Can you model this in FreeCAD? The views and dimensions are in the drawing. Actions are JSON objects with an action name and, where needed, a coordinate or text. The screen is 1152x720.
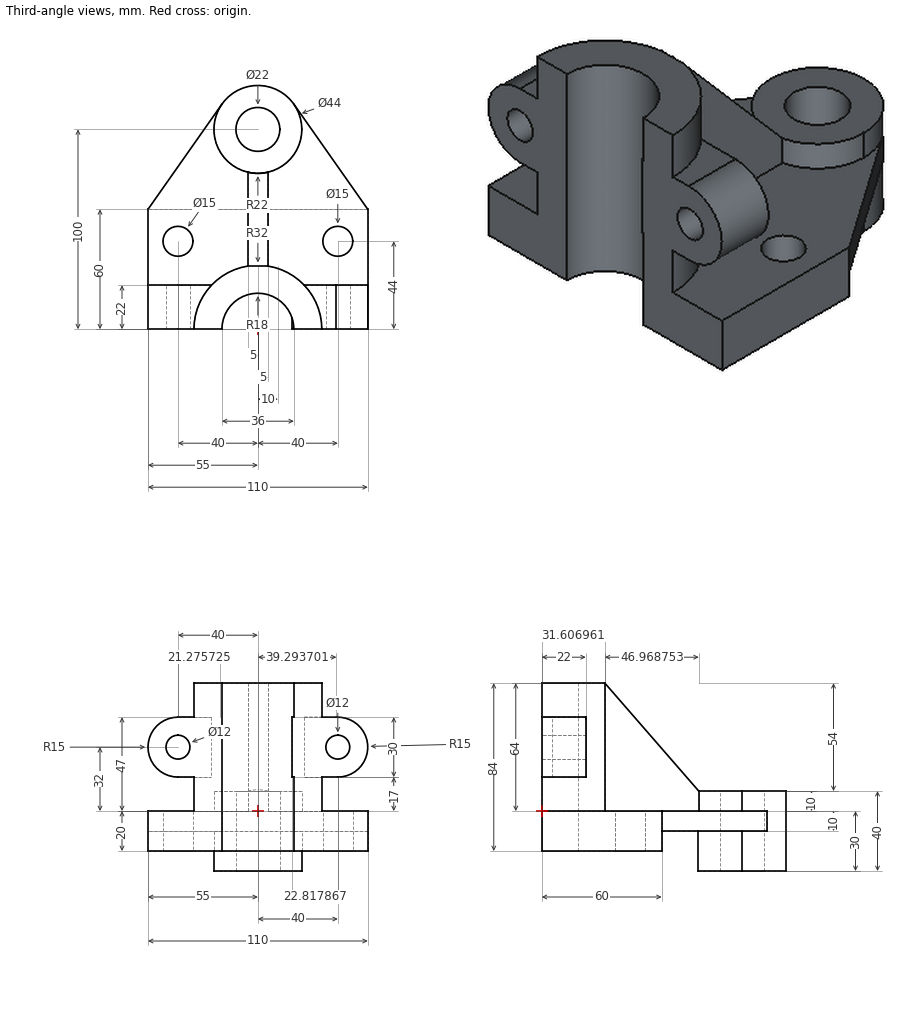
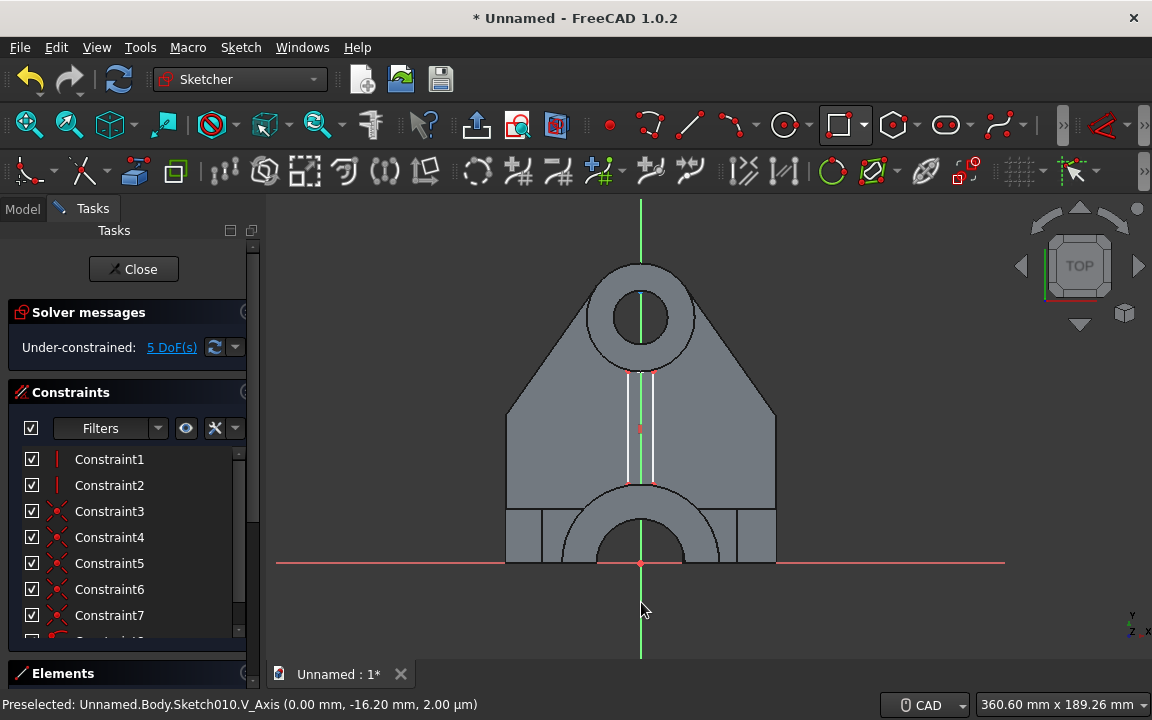
{"action": "left_click", "coordinate": [1102, 126]}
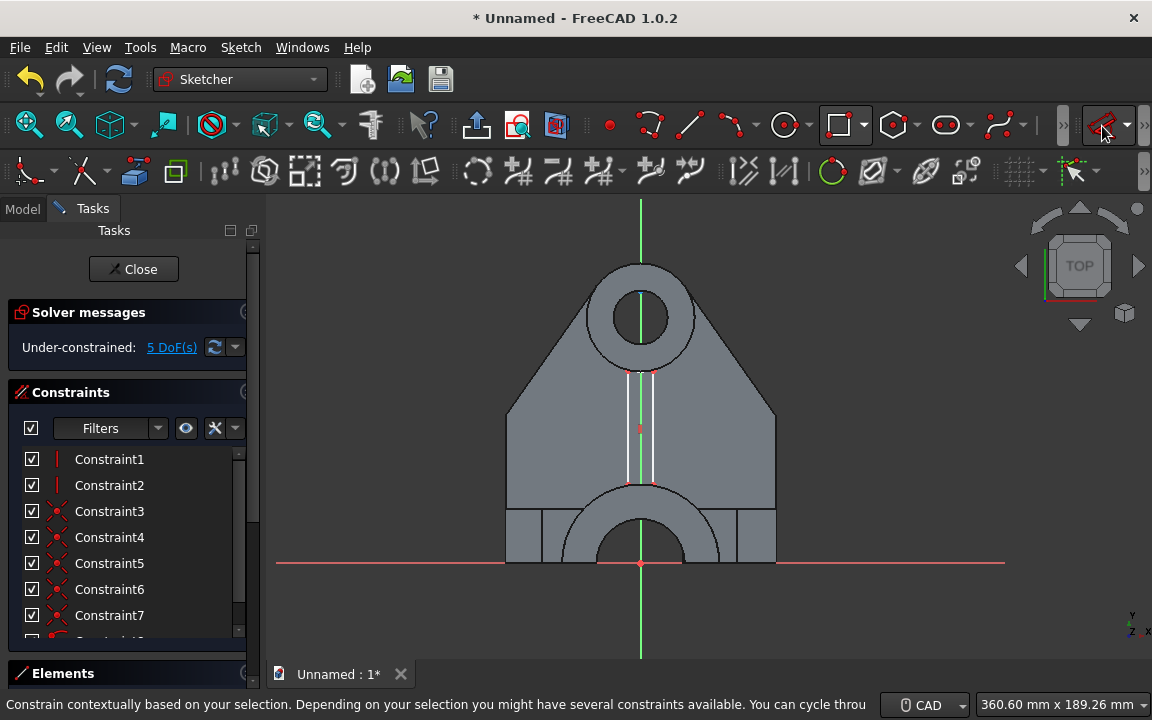
{"action": "left_click", "coordinate": [641, 485]}
{"action": "left_click", "coordinate": [694, 467]}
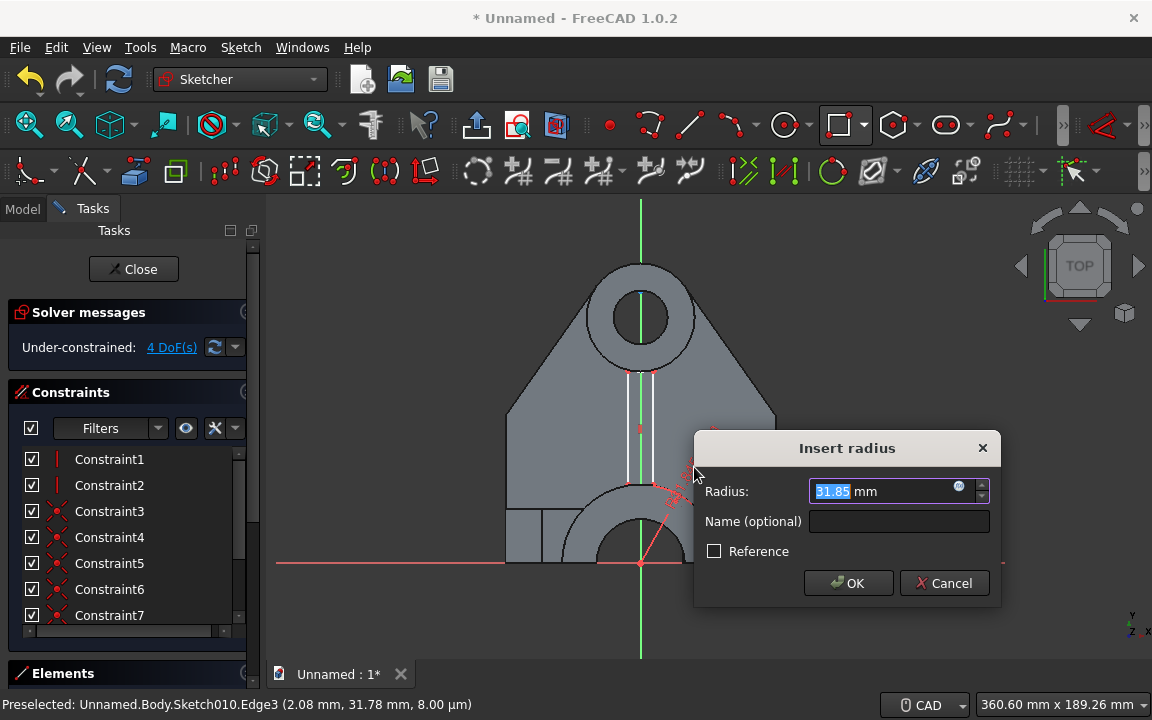
{"action": "type", "text": "32"}
{"action": "key", "text": "Return"}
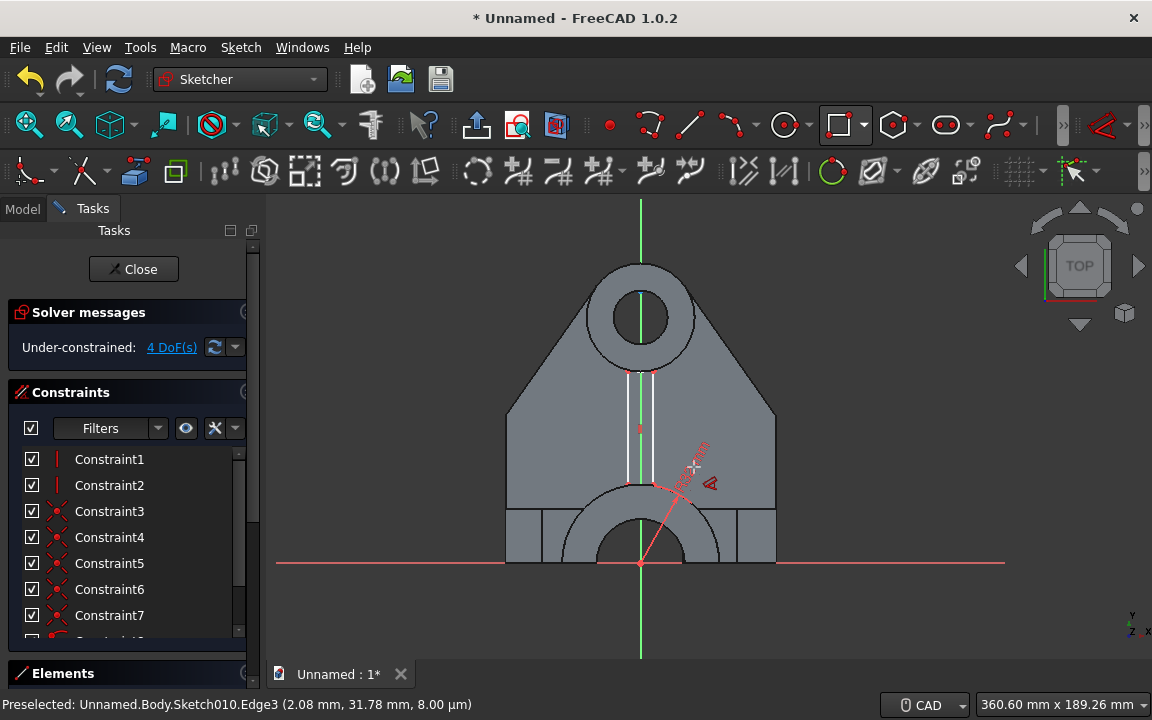
{"action": "left_click", "coordinate": [641, 372]}
{"action": "left_click", "coordinate": [587, 390]}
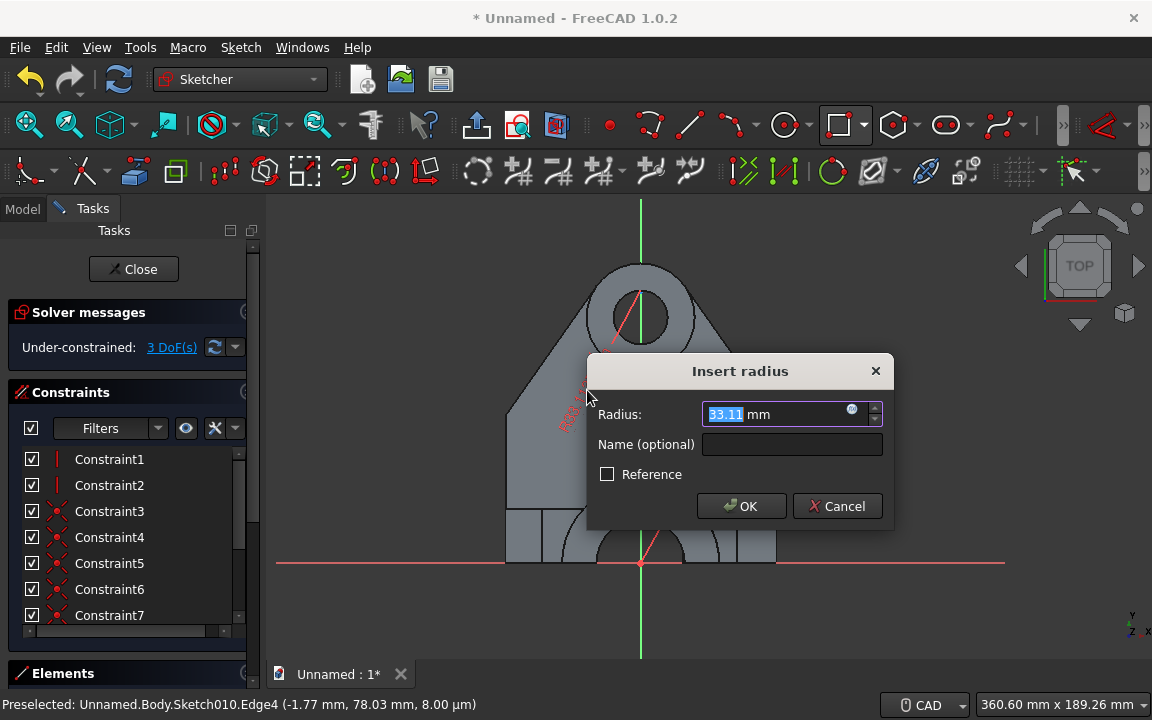
{"action": "type", "text": "22"}
{"action": "key", "text": "Return"}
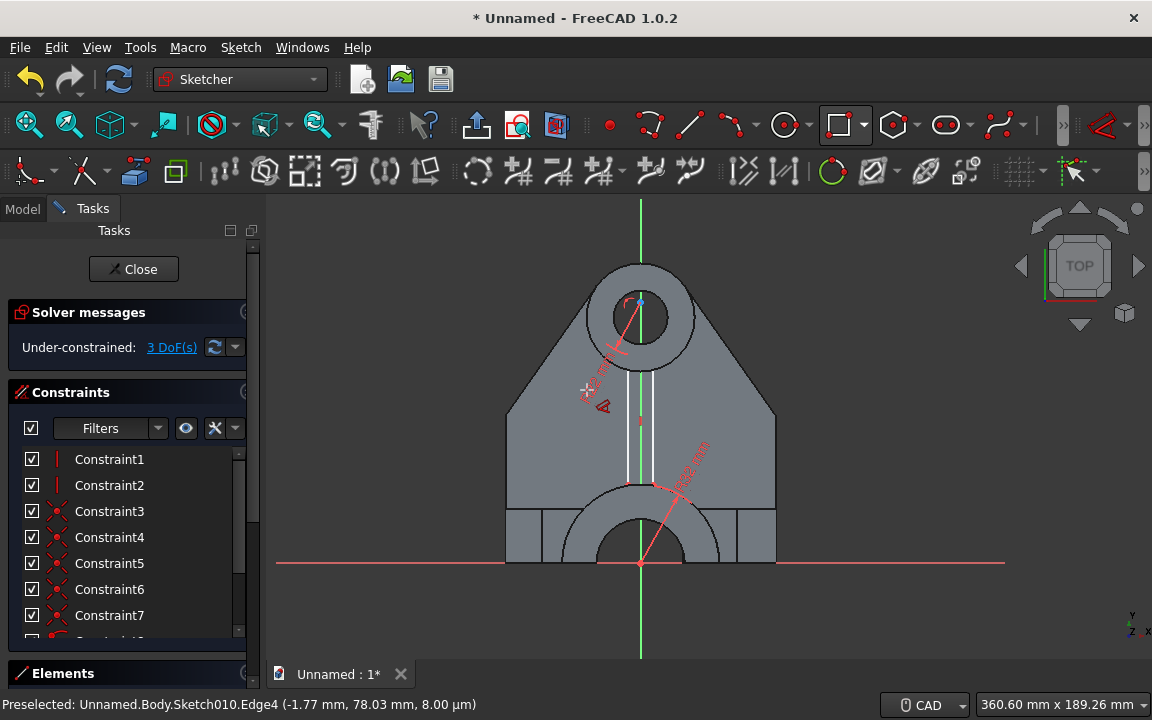
{"action": "scroll", "coordinate": [628, 355], "scroll_direction": "up", "scroll_amount": 6}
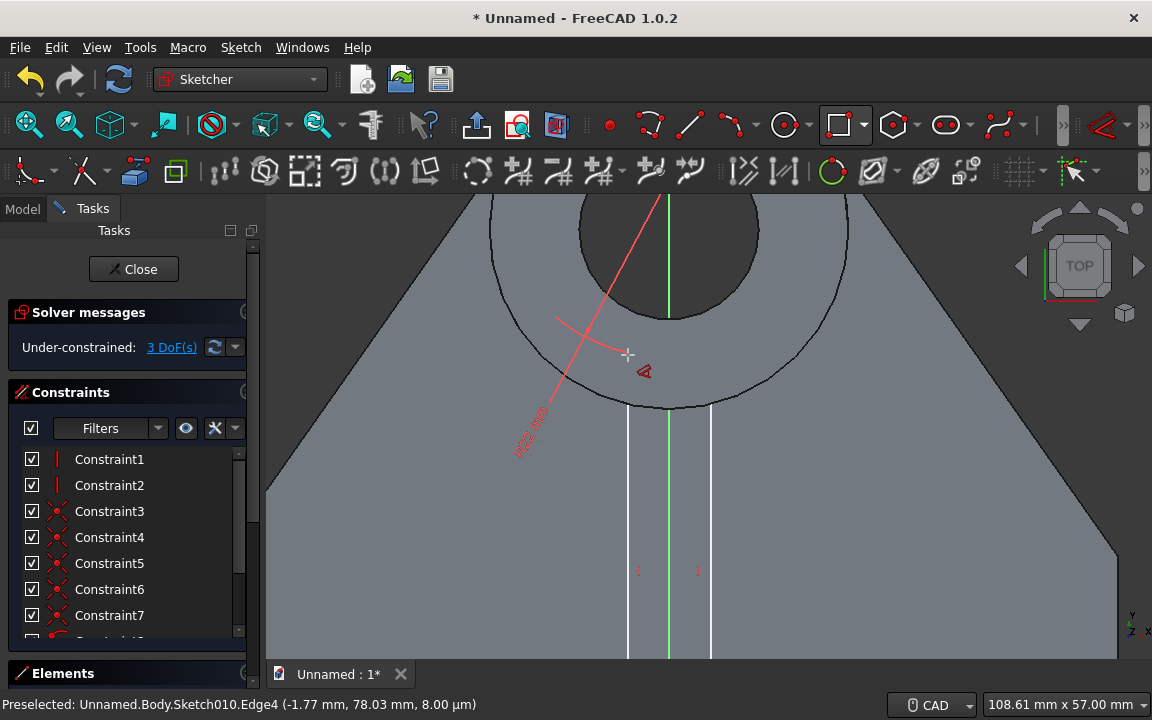
{"action": "left_click", "coordinate": [628, 353]}
{"action": "left_click", "coordinate": [649, 319]}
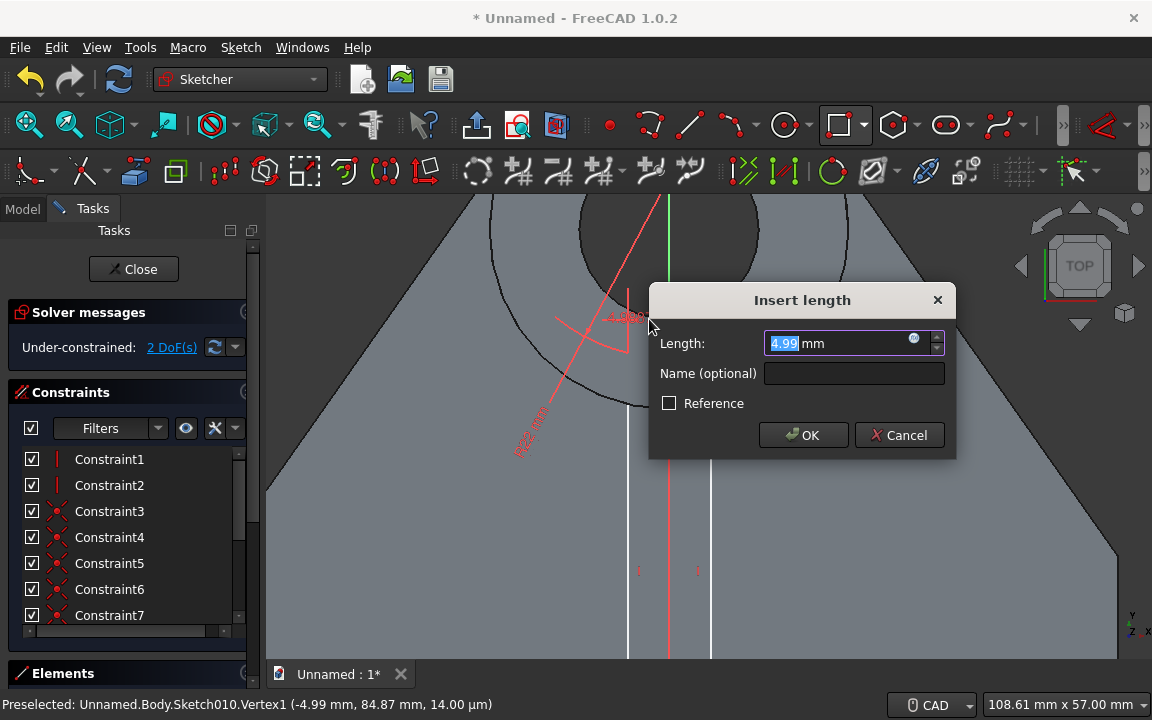
{"action": "type", "text": "5"}
{"action": "key", "text": "Return"}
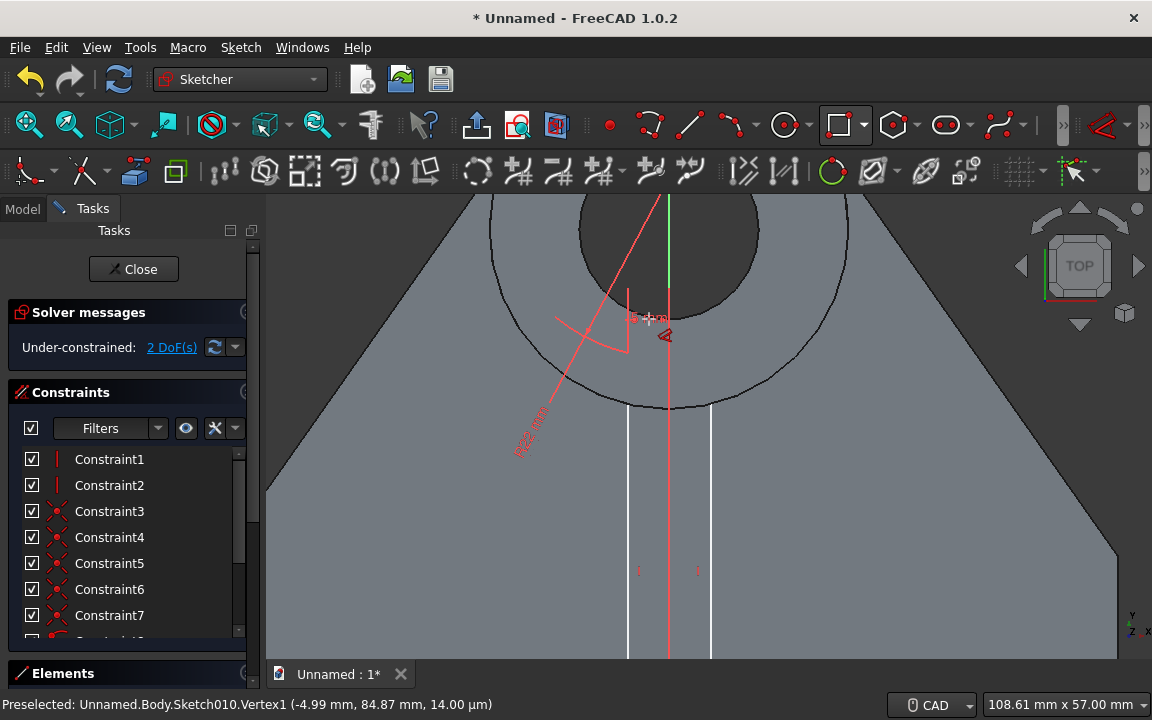
{"action": "scroll", "coordinate": [617, 222], "scroll_direction": "down", "scroll_amount": 4}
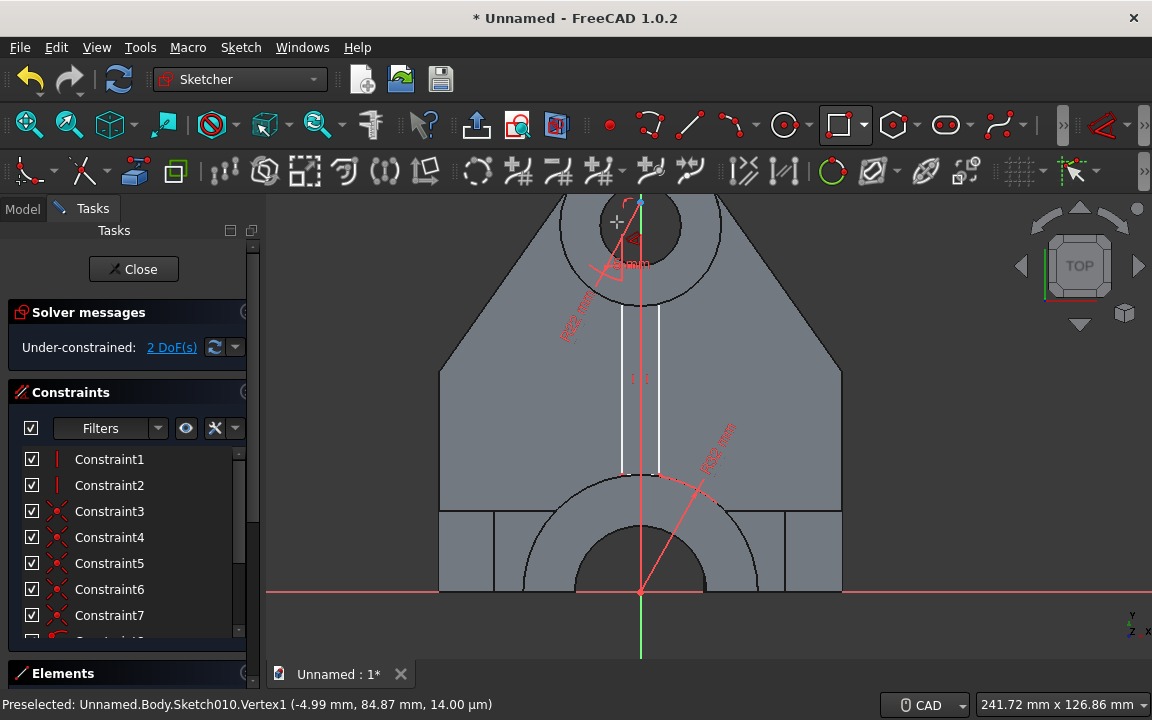
{"action": "scroll", "coordinate": [659, 476], "scroll_direction": "up", "scroll_amount": 4}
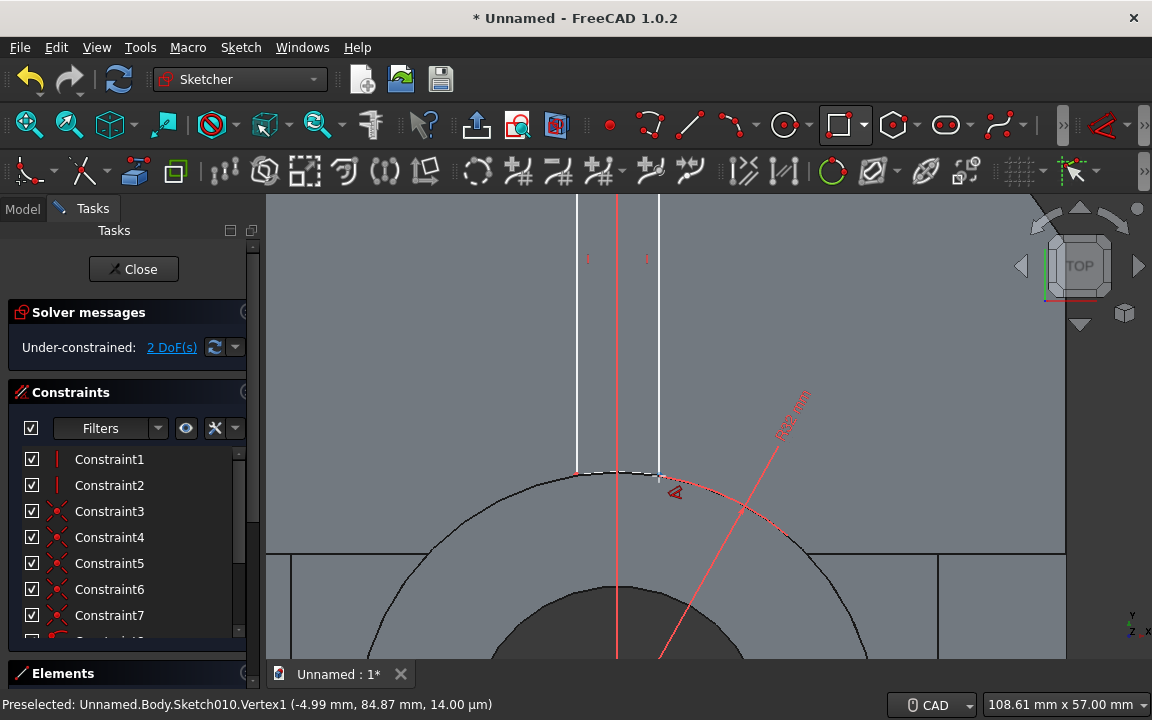
{"action": "left_click", "coordinate": [659, 476]}
{"action": "left_click", "coordinate": [638, 442]}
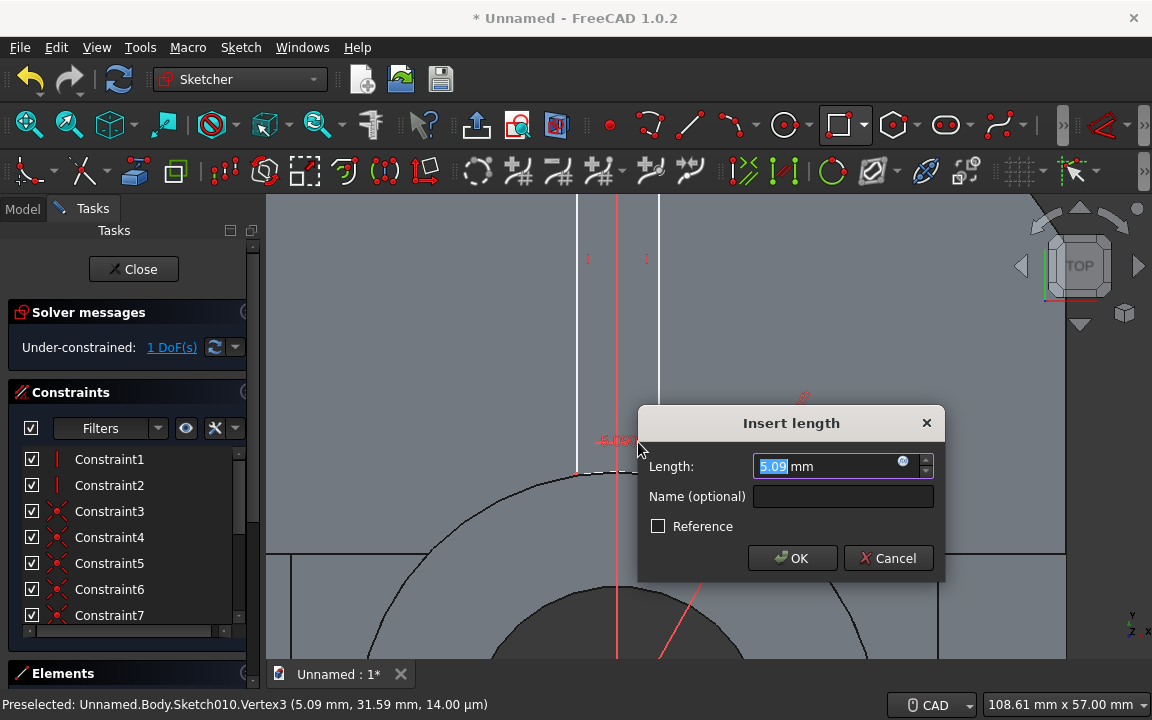
{"action": "type", "text": "5"}
{"action": "key", "text": "Return"}